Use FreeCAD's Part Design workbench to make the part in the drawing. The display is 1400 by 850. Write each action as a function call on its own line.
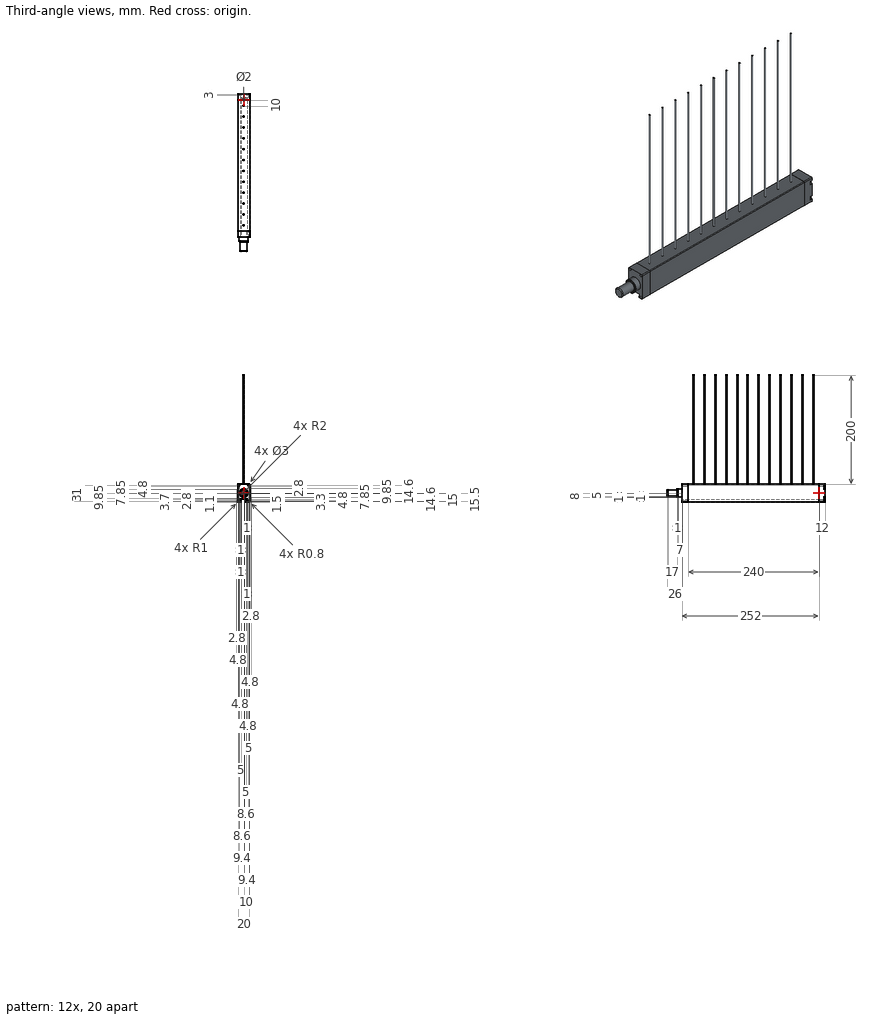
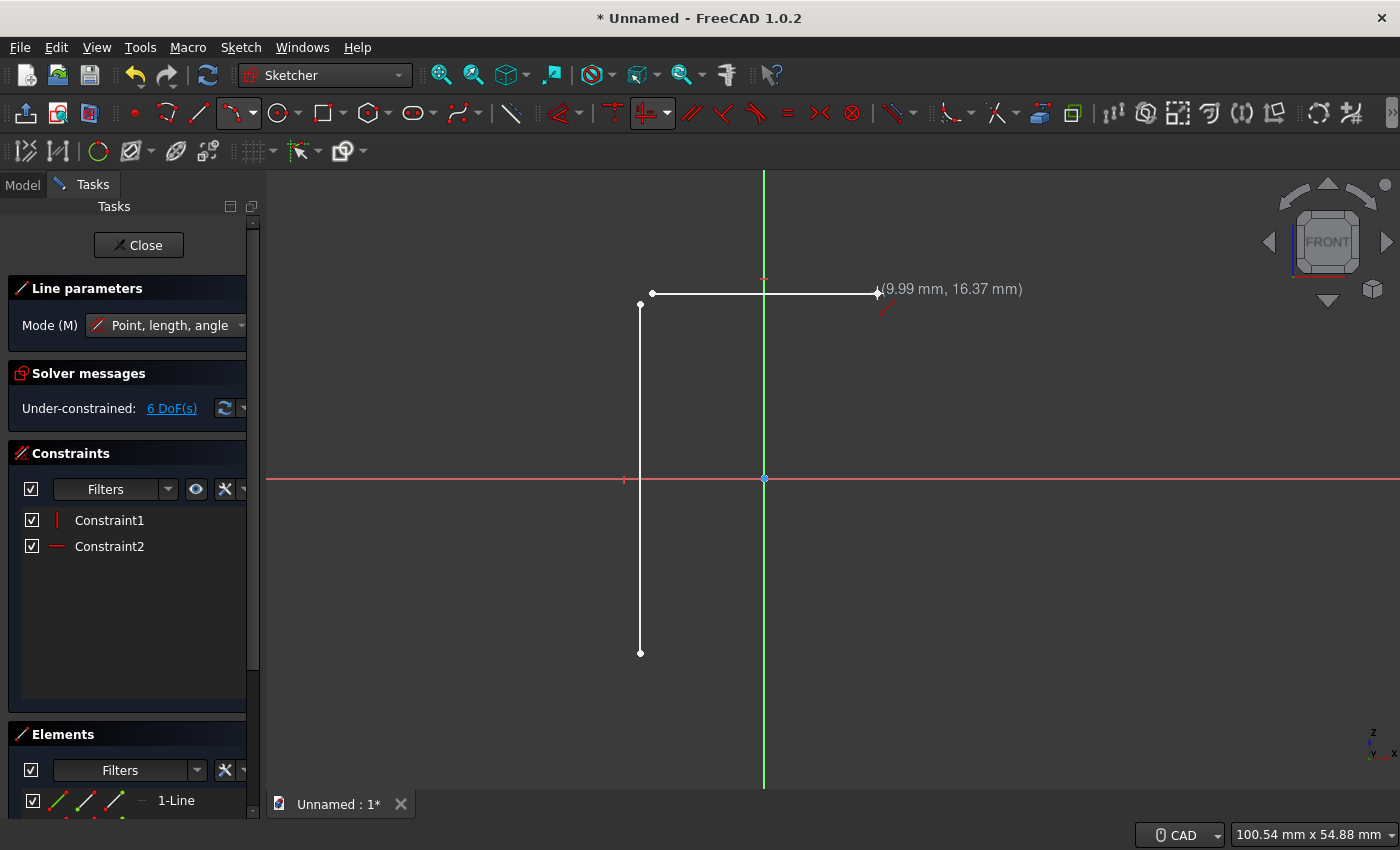
click(888, 304)
click(888, 653)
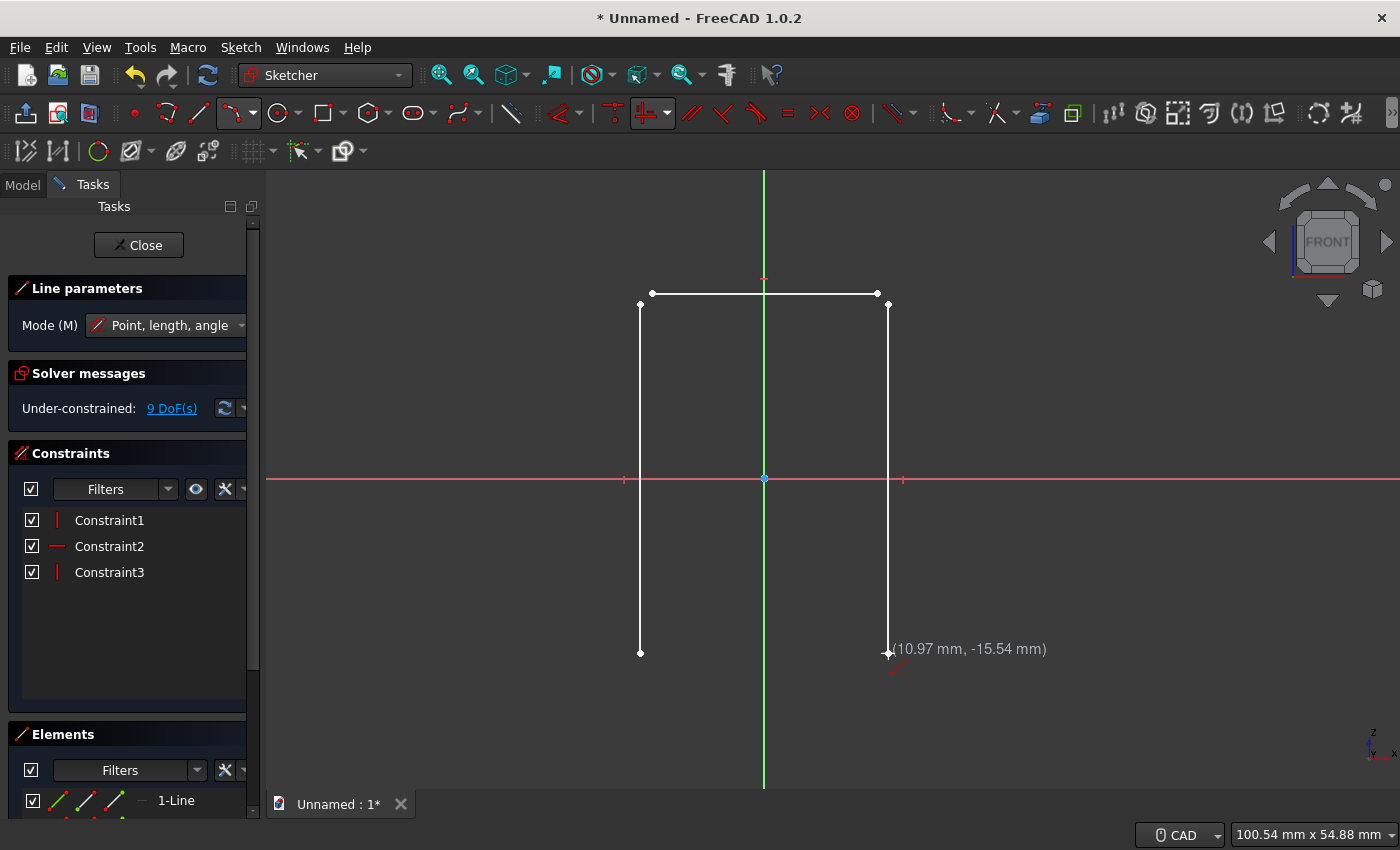
key(g)
key(m)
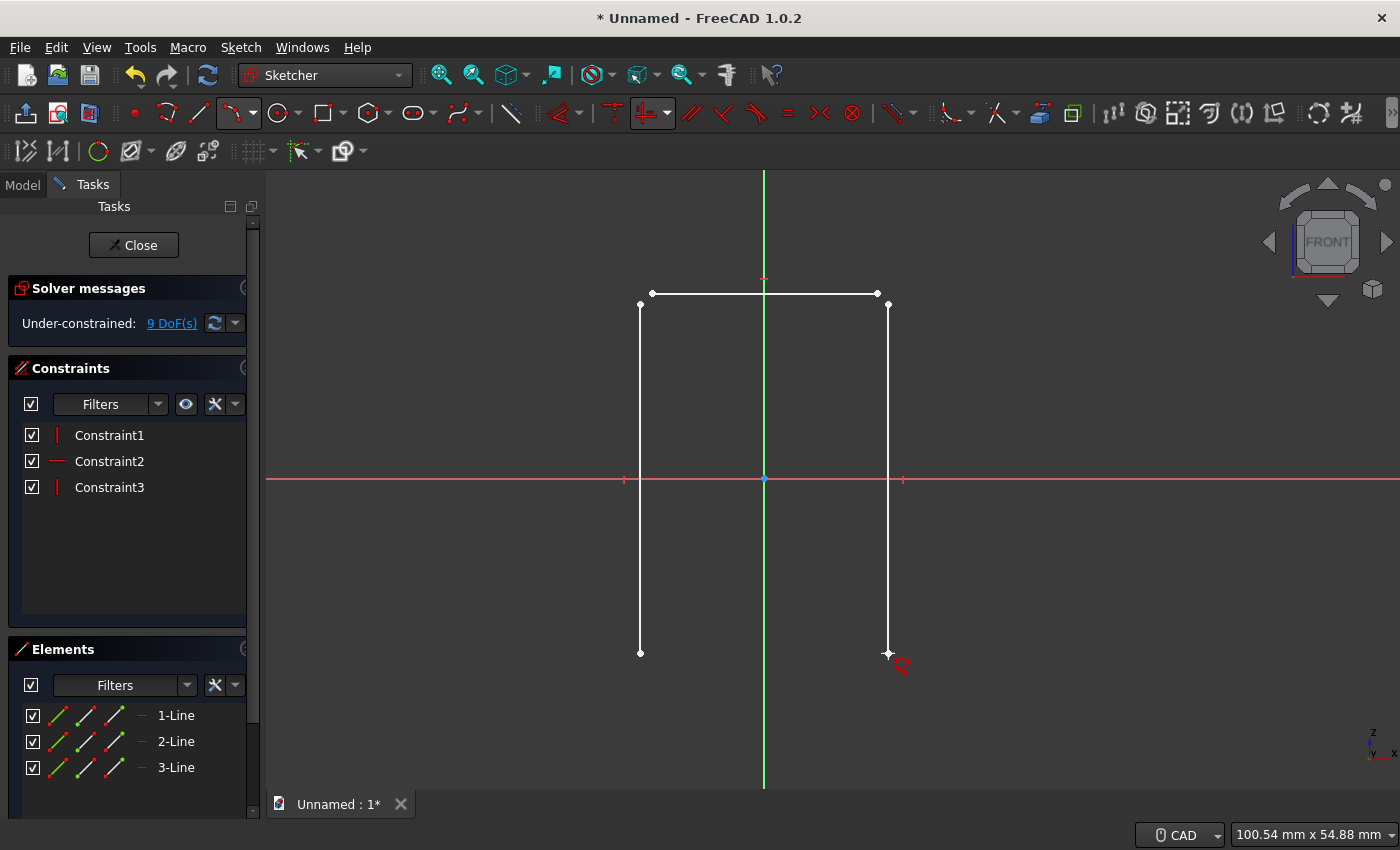
click(877, 665)
click(821, 665)
click(821, 648)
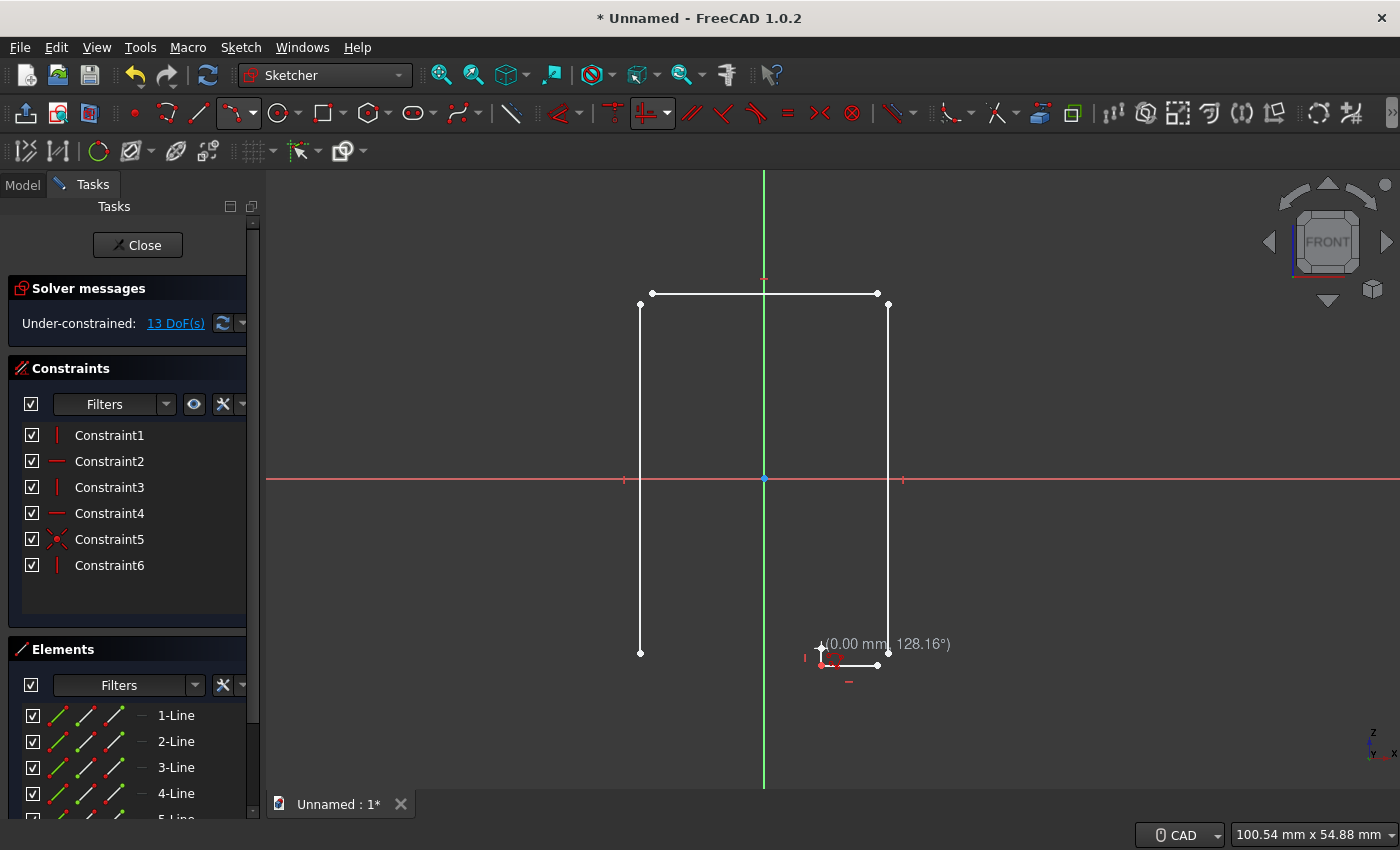
scroll(832, 648, up, 2)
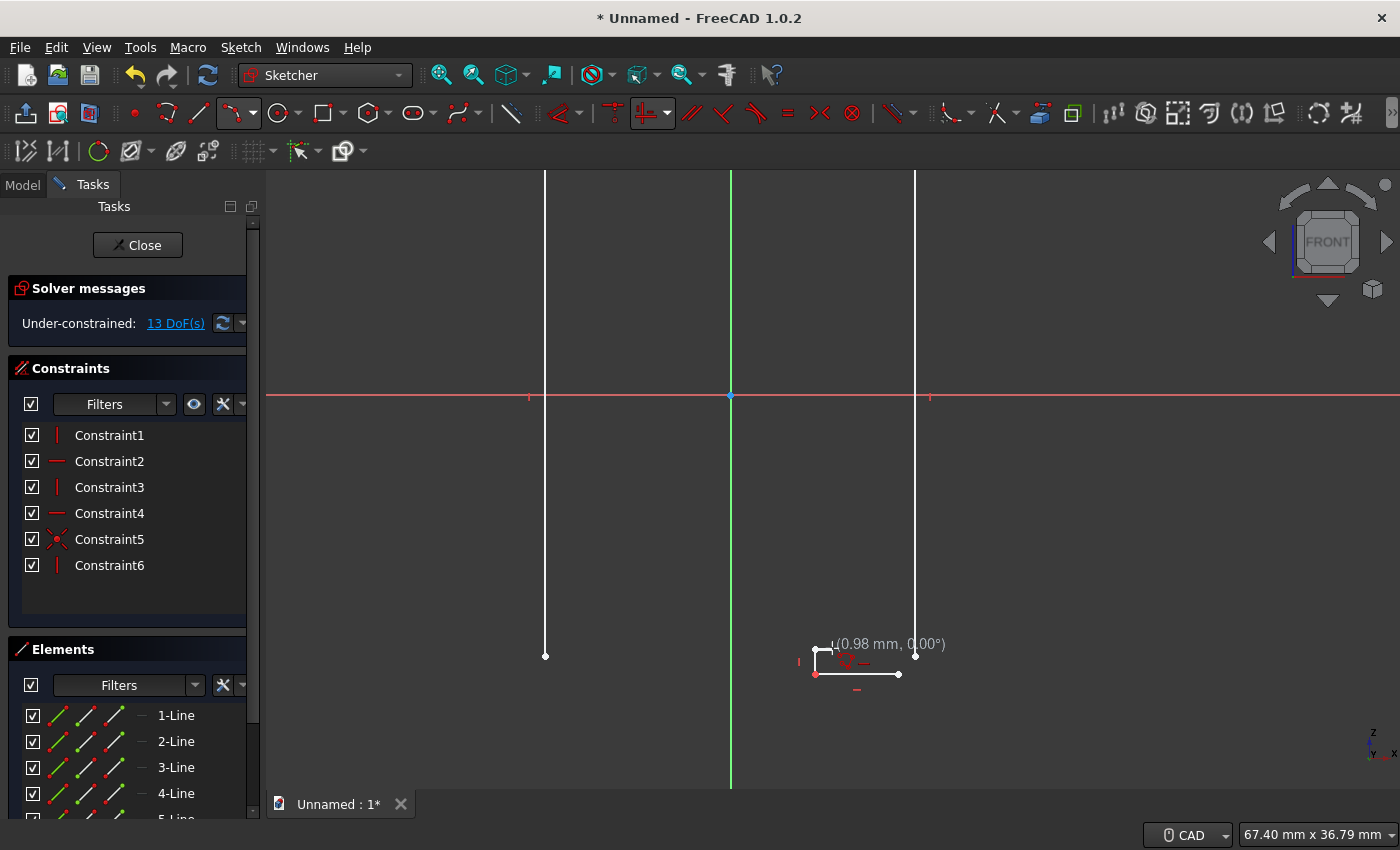
click(832, 648)
click(832, 592)
click(630, 592)
click(630, 647)
click(647, 647)
click(647, 673)
click(562, 673)
right_click(562, 673)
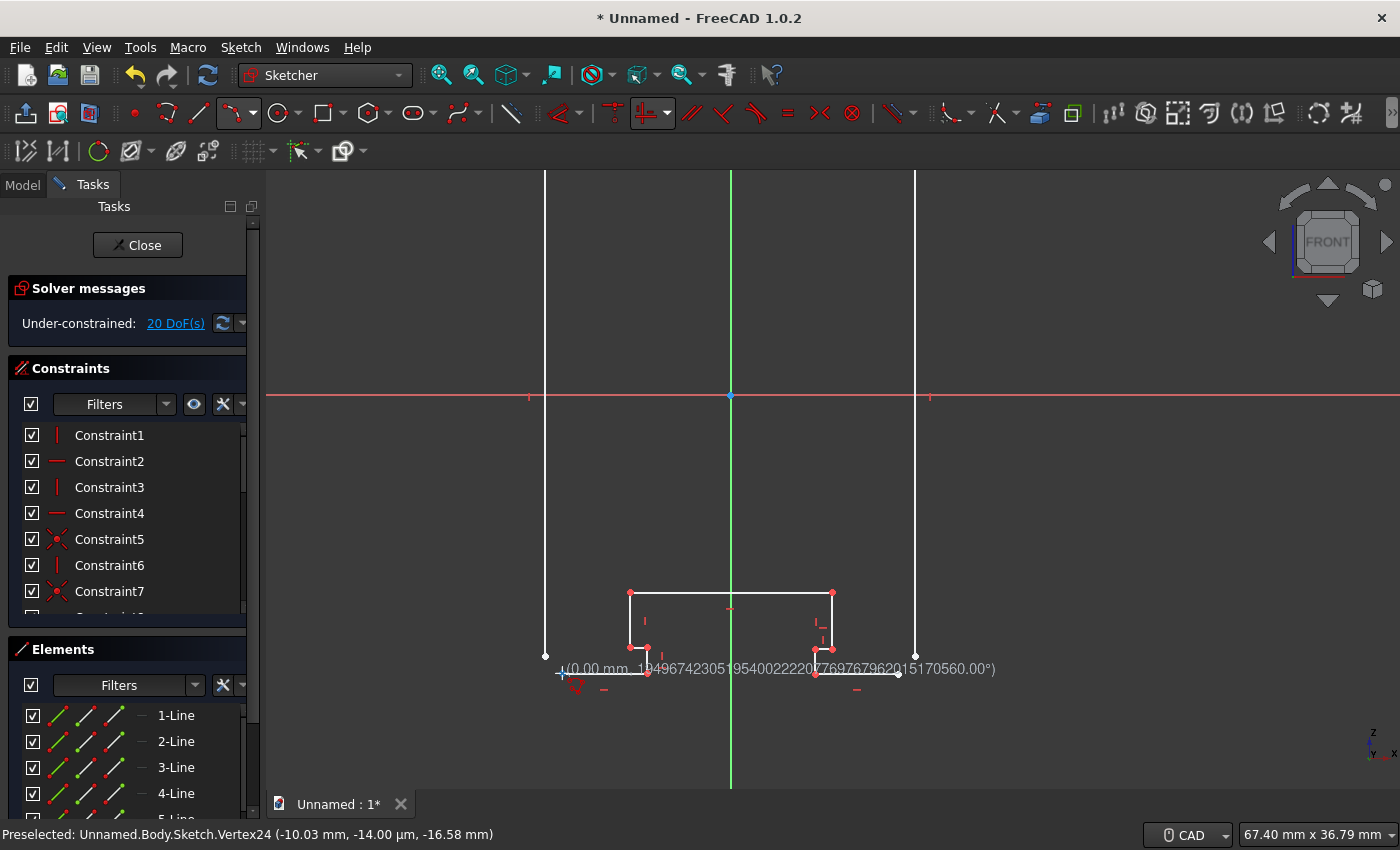
click(232, 114)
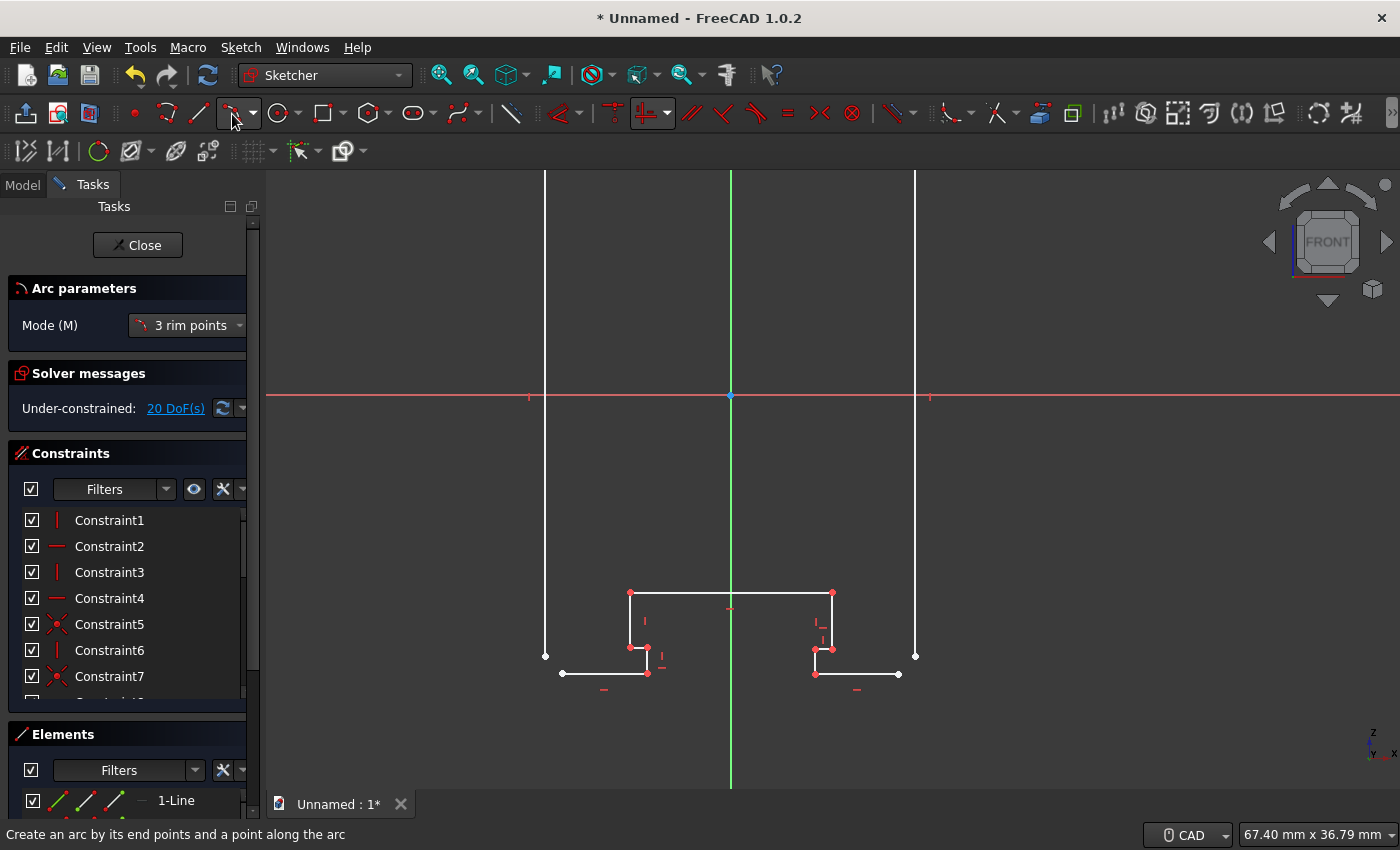
scroll(833, 651, down, 2)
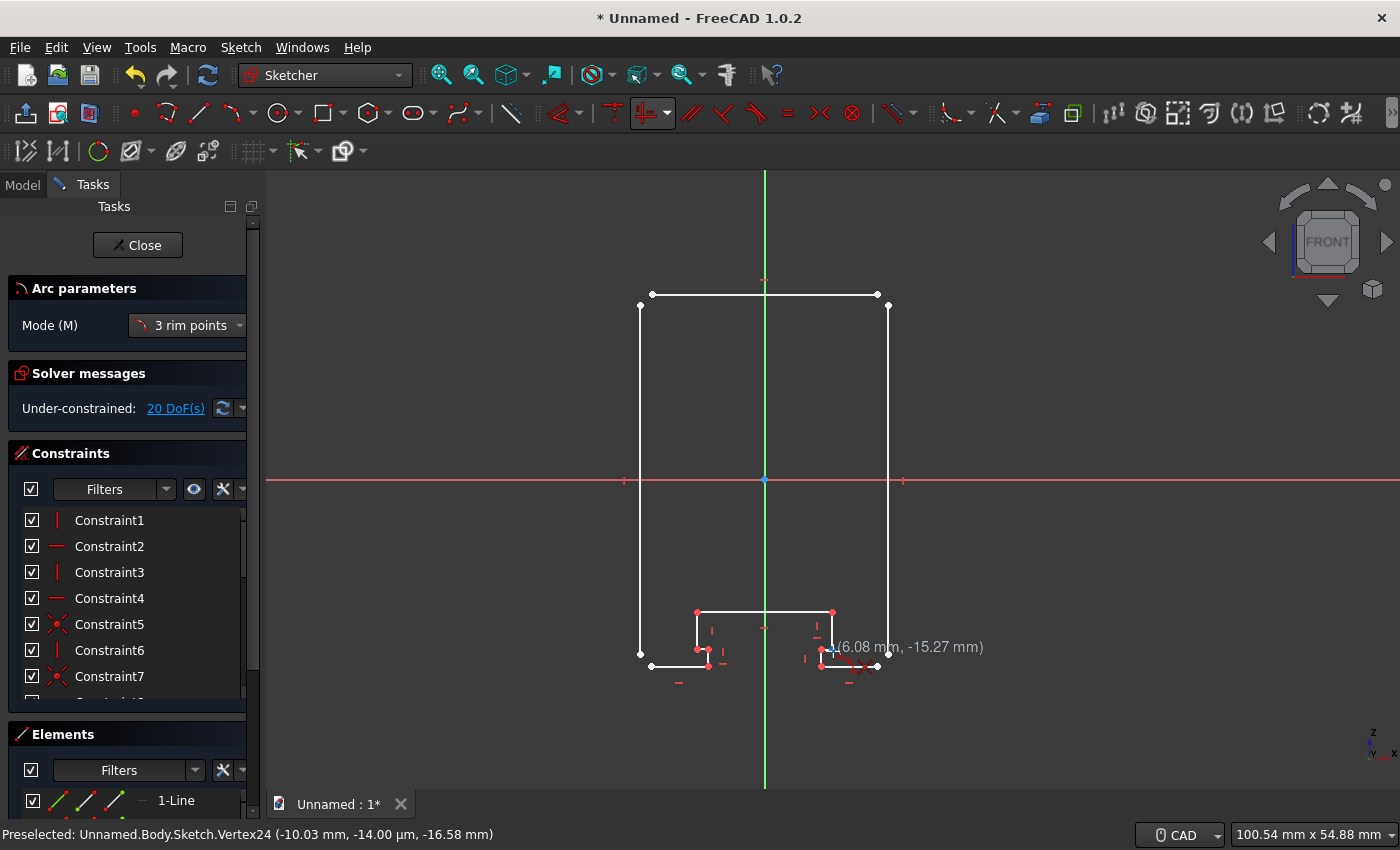
click(640, 306)
click(652, 295)